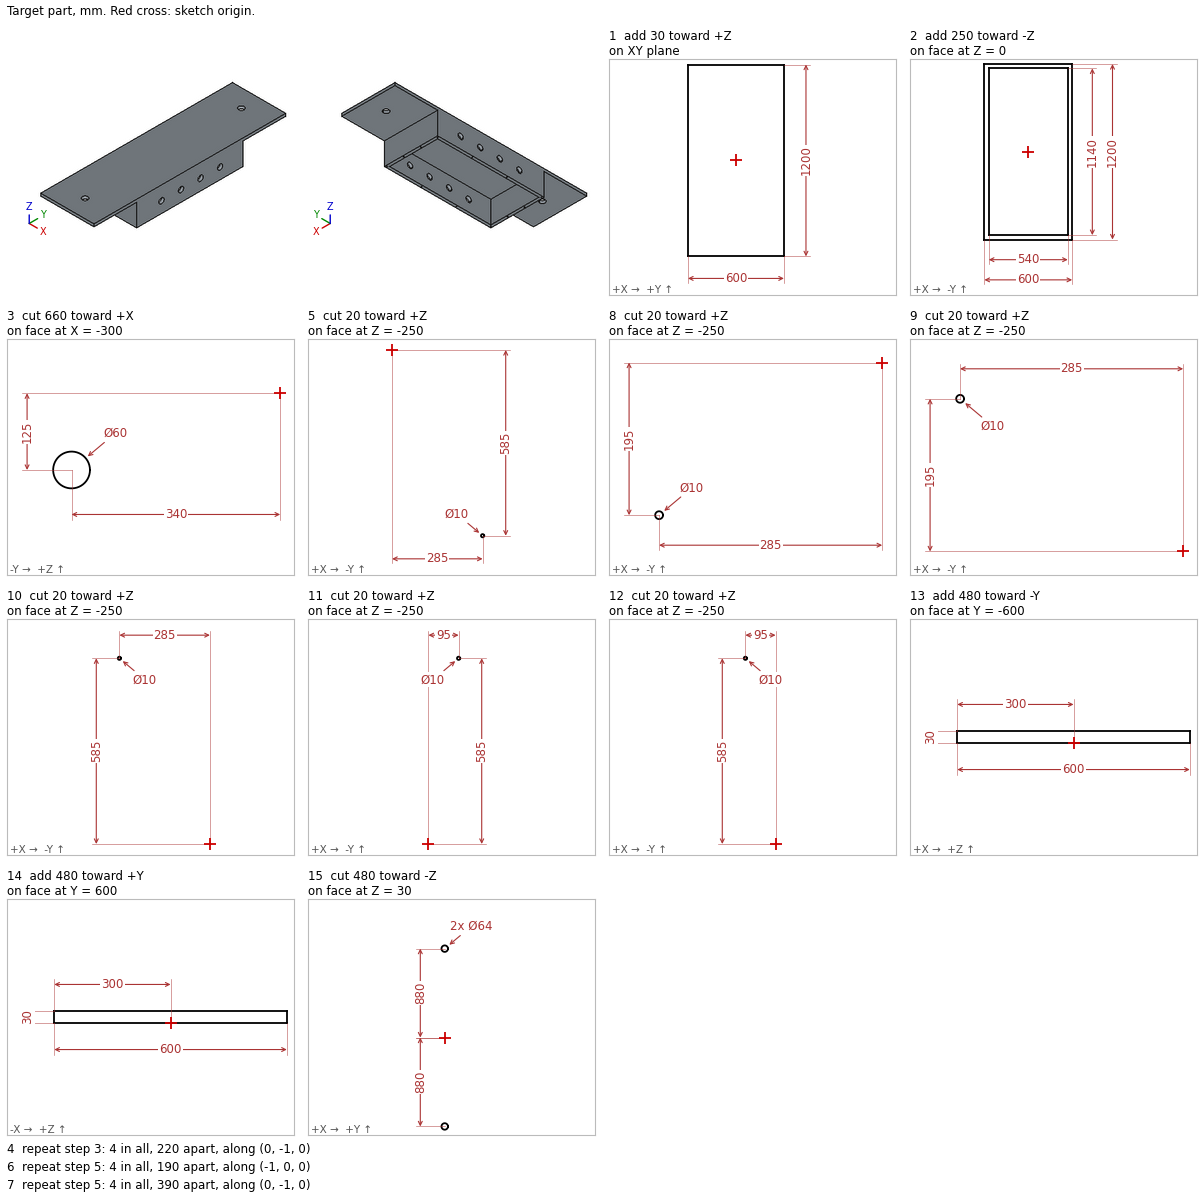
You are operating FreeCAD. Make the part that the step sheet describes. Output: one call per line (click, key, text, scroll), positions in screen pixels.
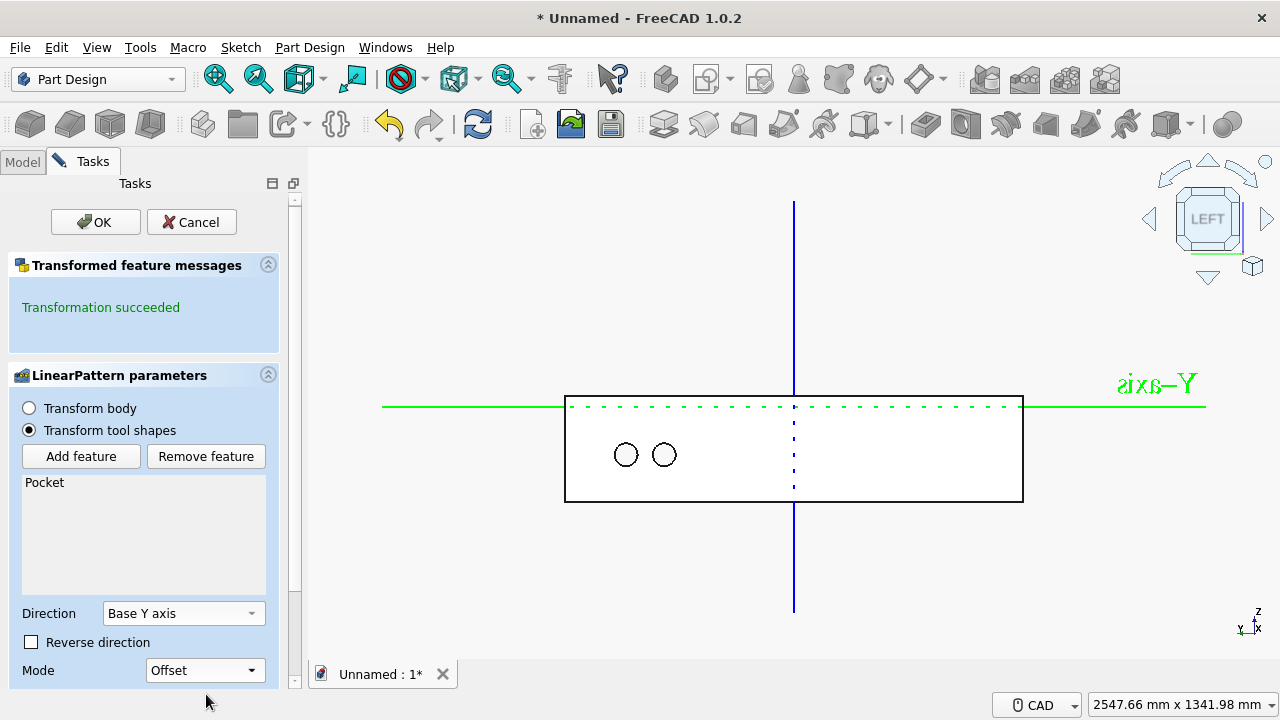
scroll(295, 440, down, 2)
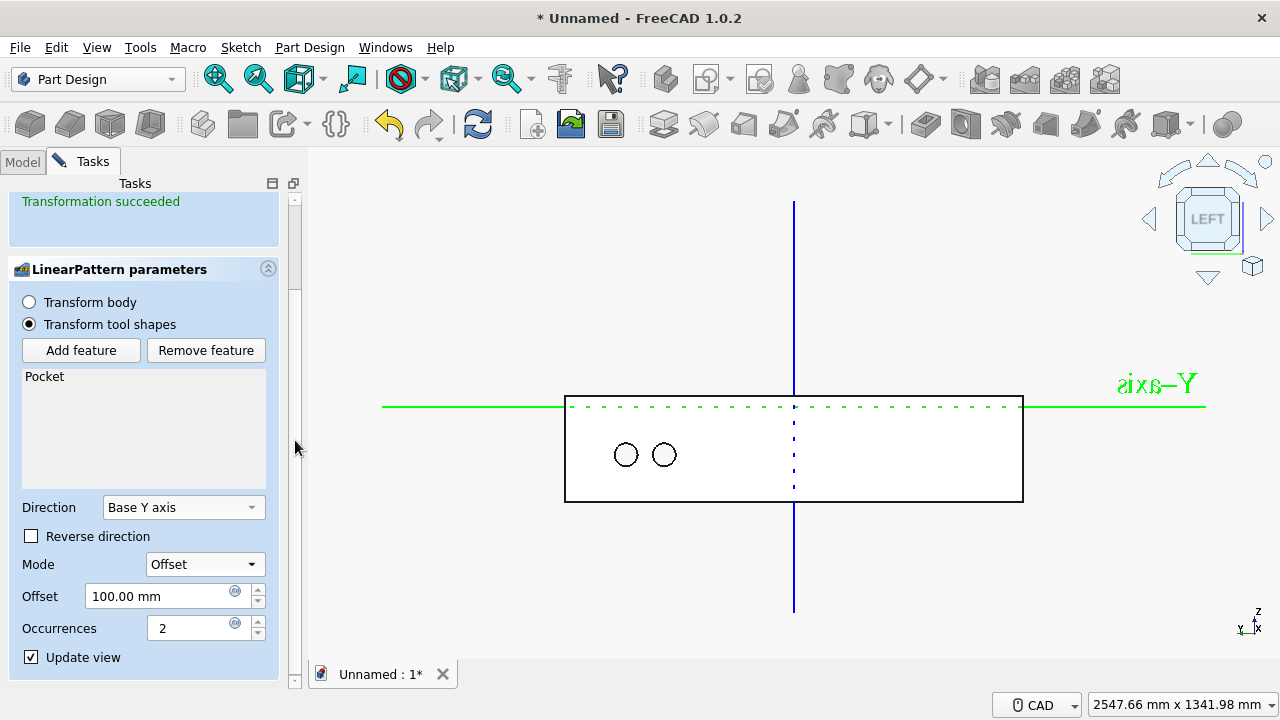
triple_click(168, 596)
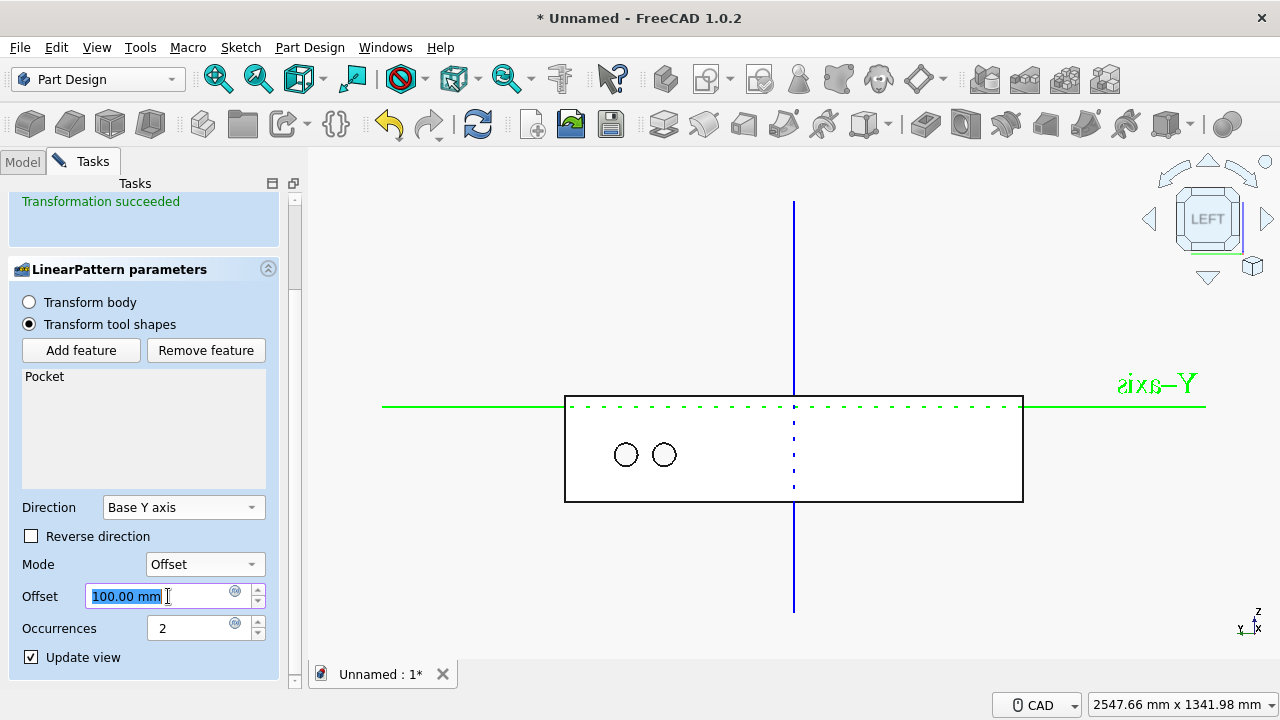
text(220)
key(Tab)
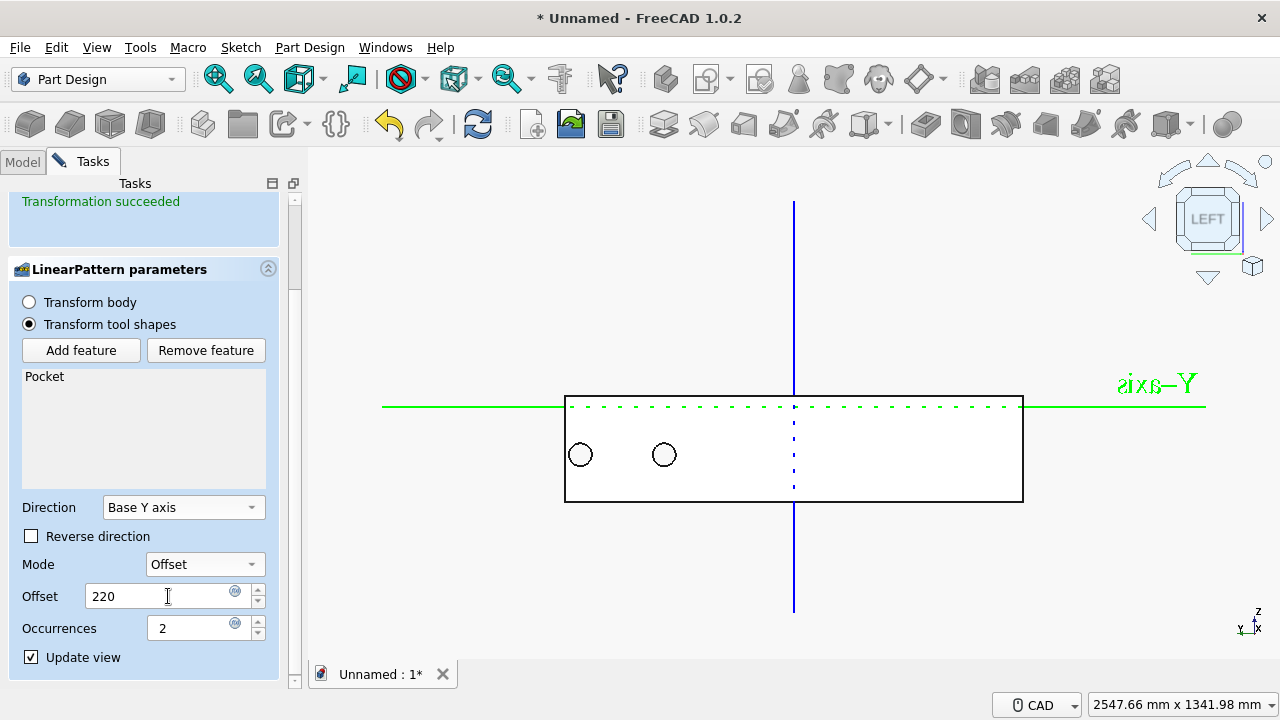
triple_click(198, 628)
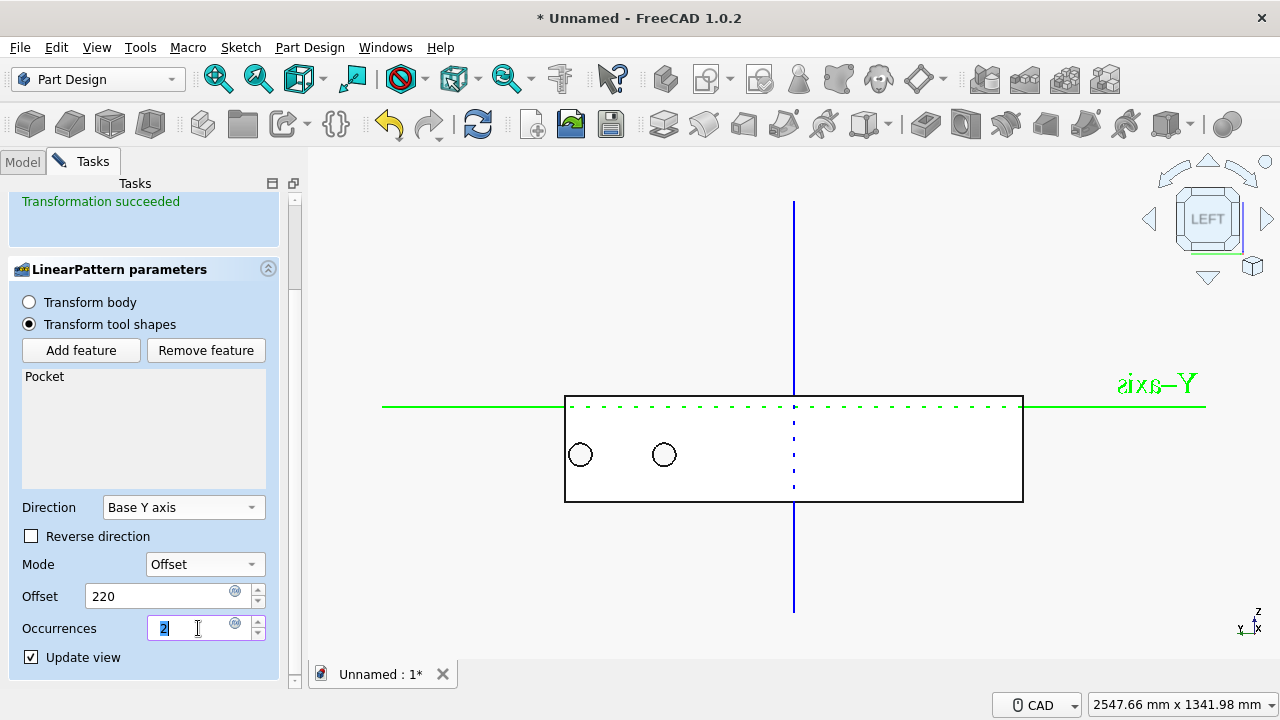
text(4)
key(Tab)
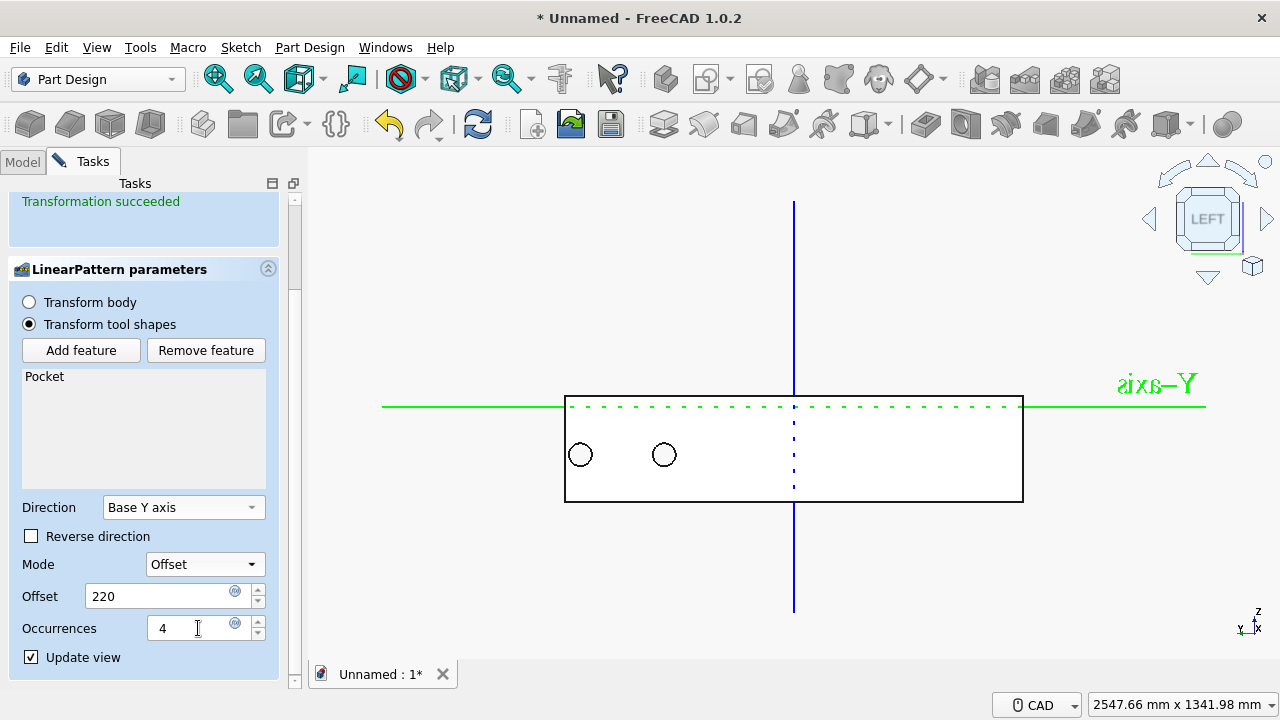
click(30, 536)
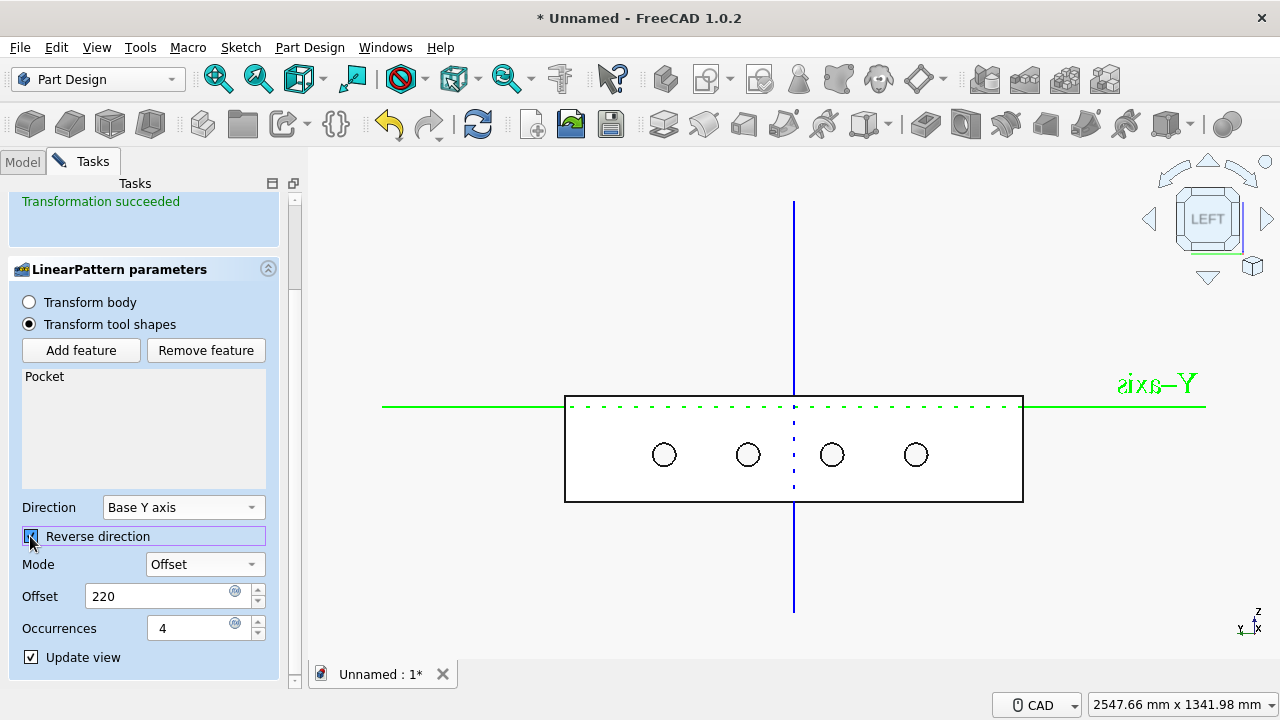
scroll(295, 440, up, 3)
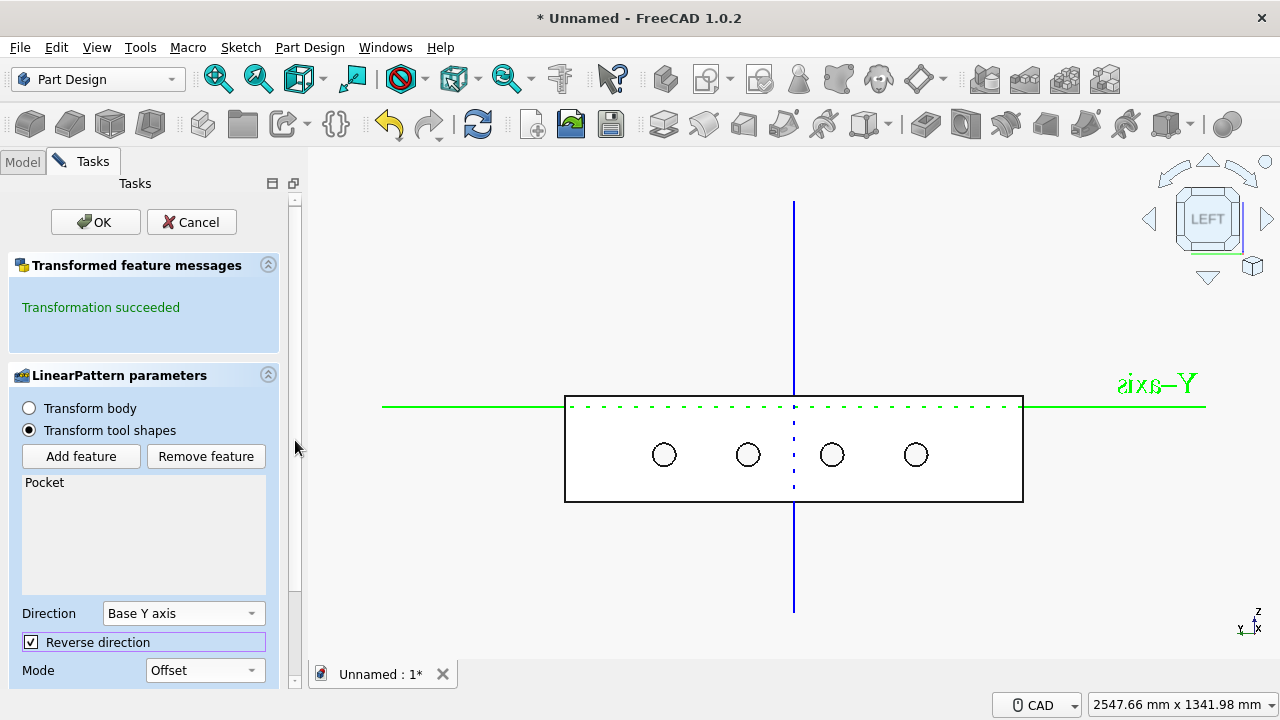
click(96, 222)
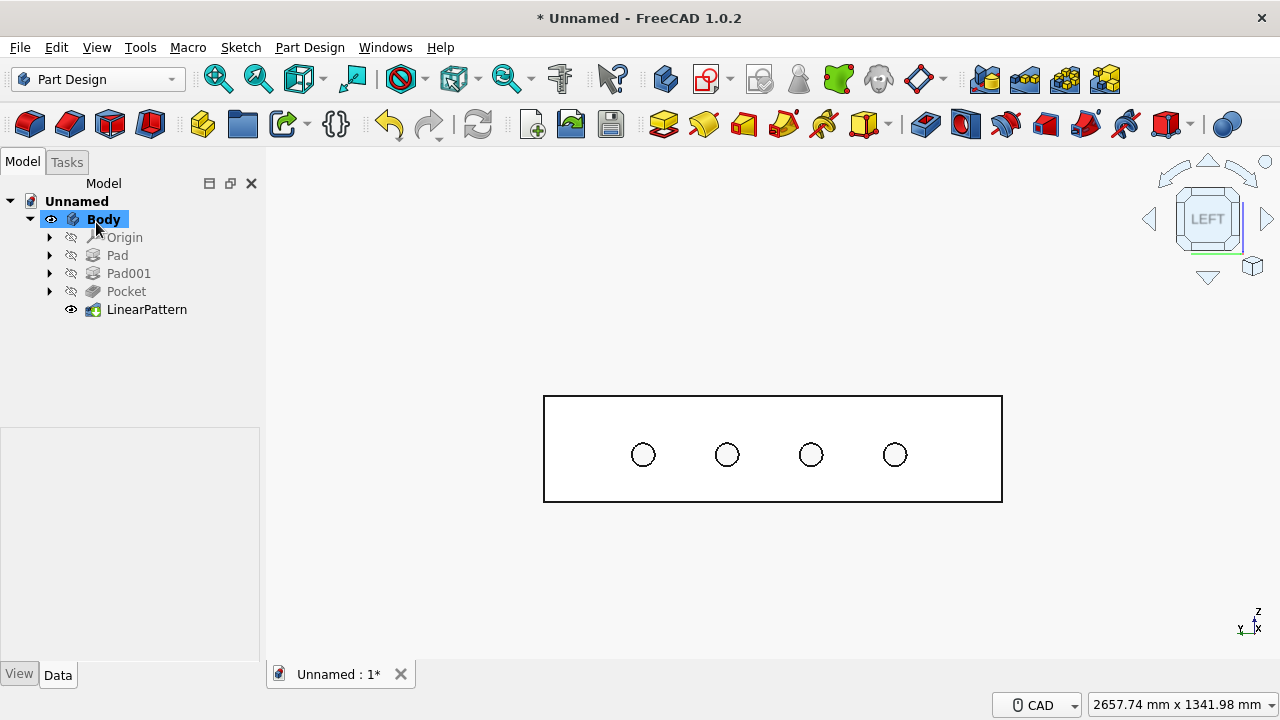
key(5)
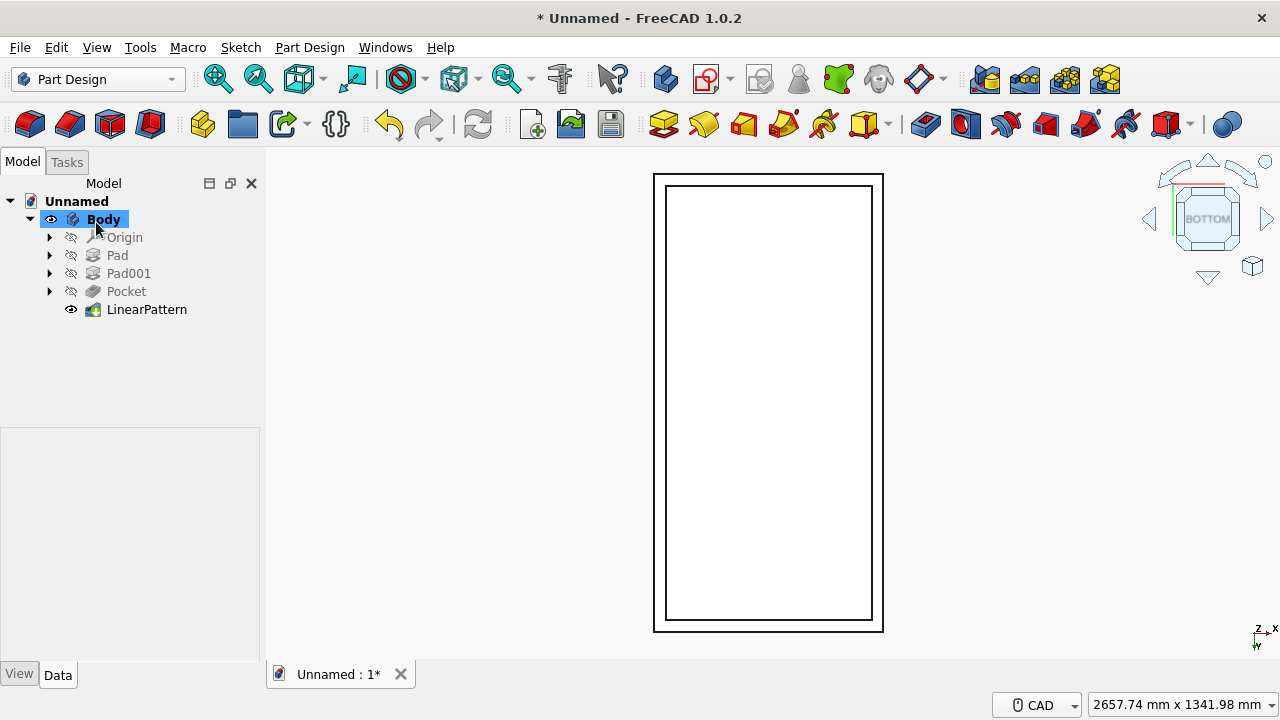
scroll(880, 474, up, 6)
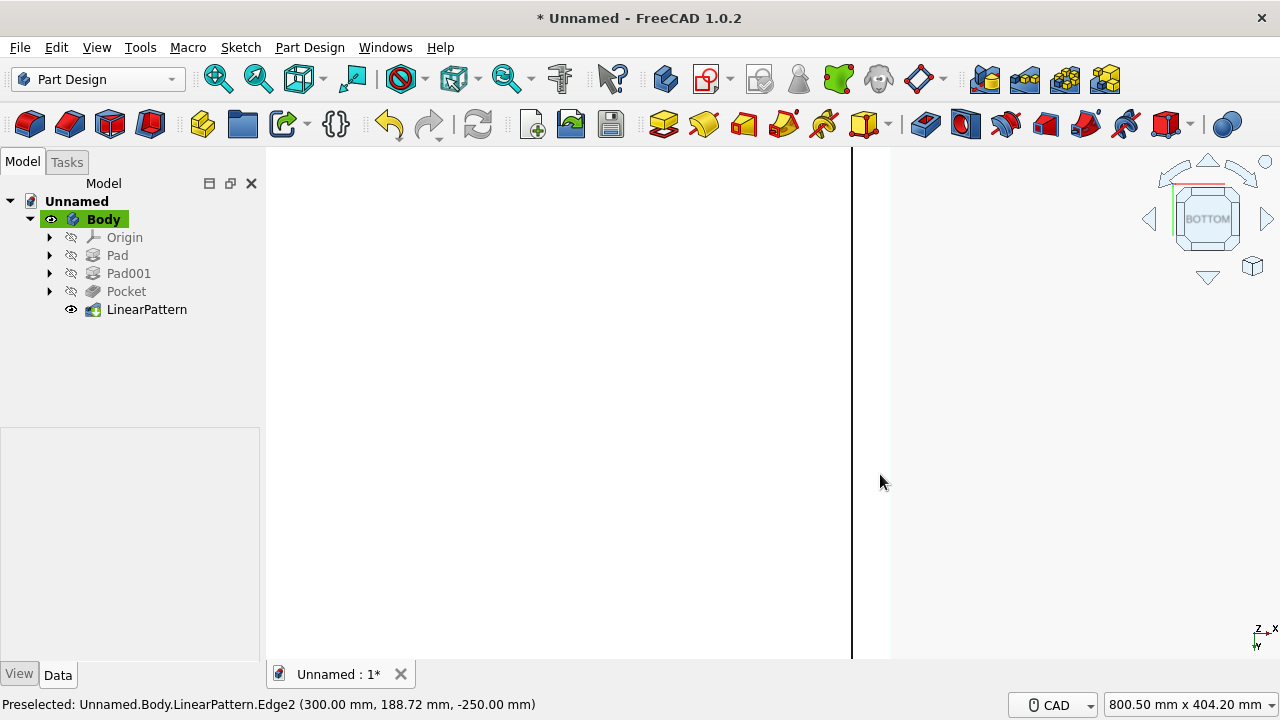
click(877, 476)